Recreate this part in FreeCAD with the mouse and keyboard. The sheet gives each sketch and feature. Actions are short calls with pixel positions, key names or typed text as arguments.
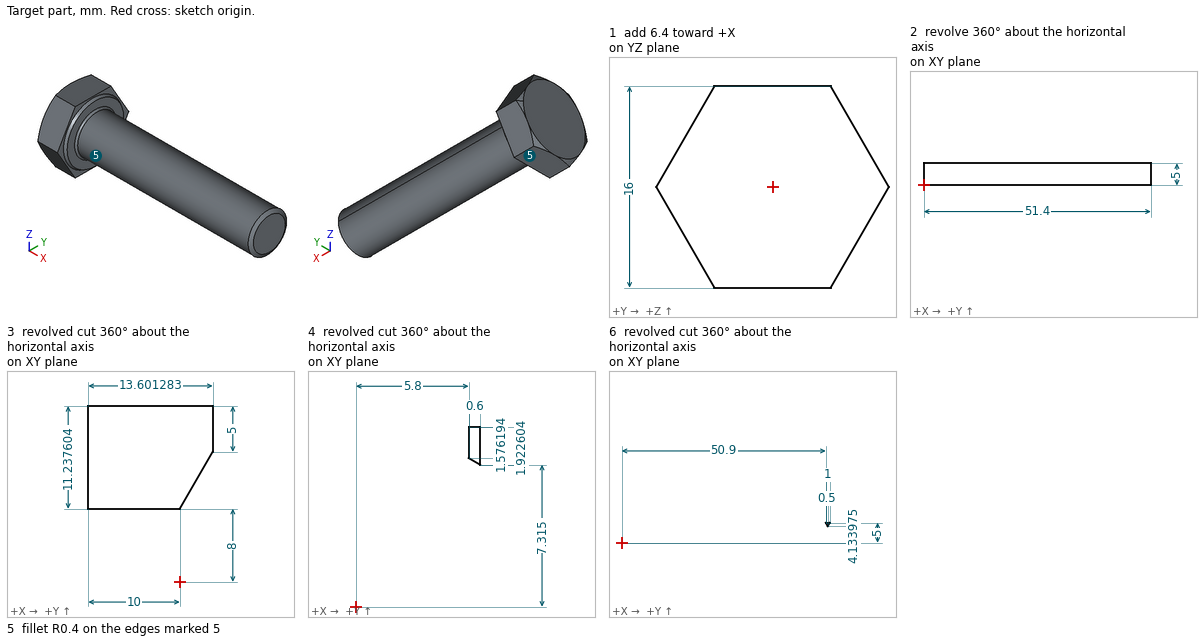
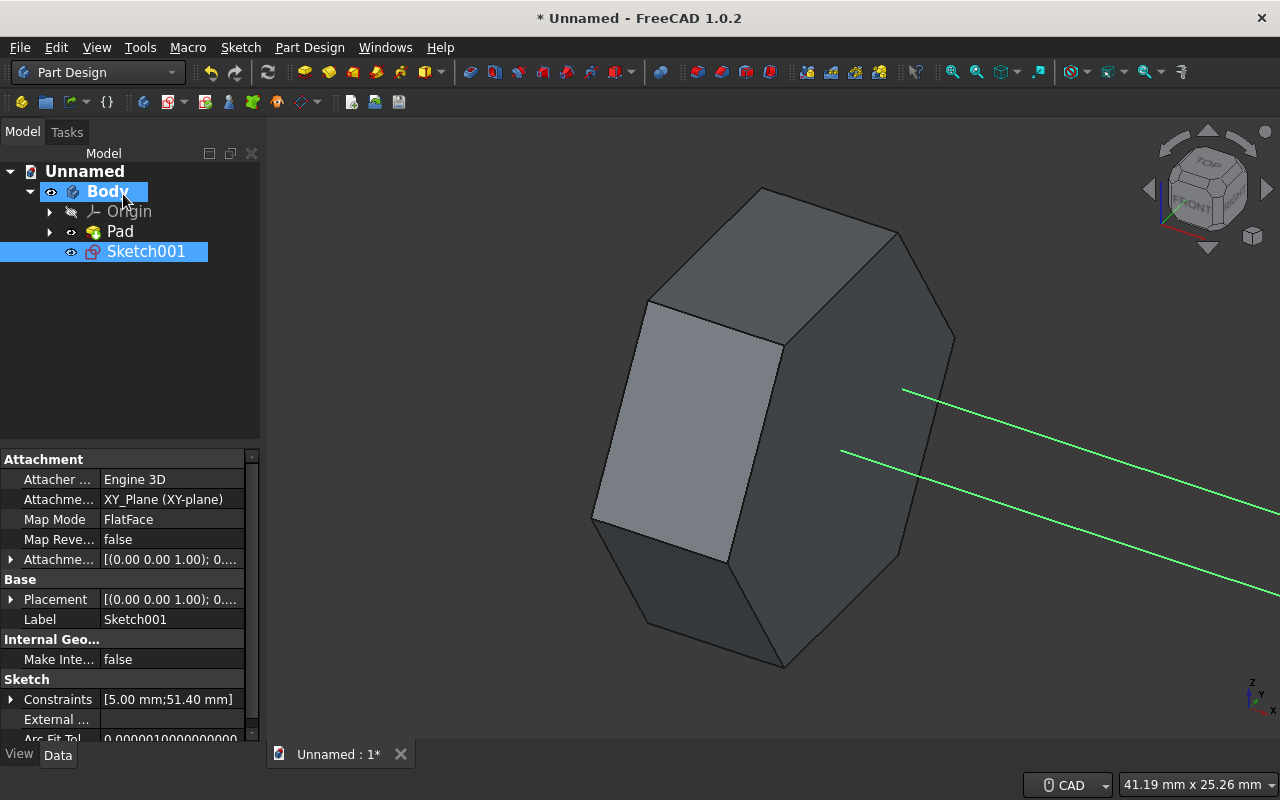
click(330, 72)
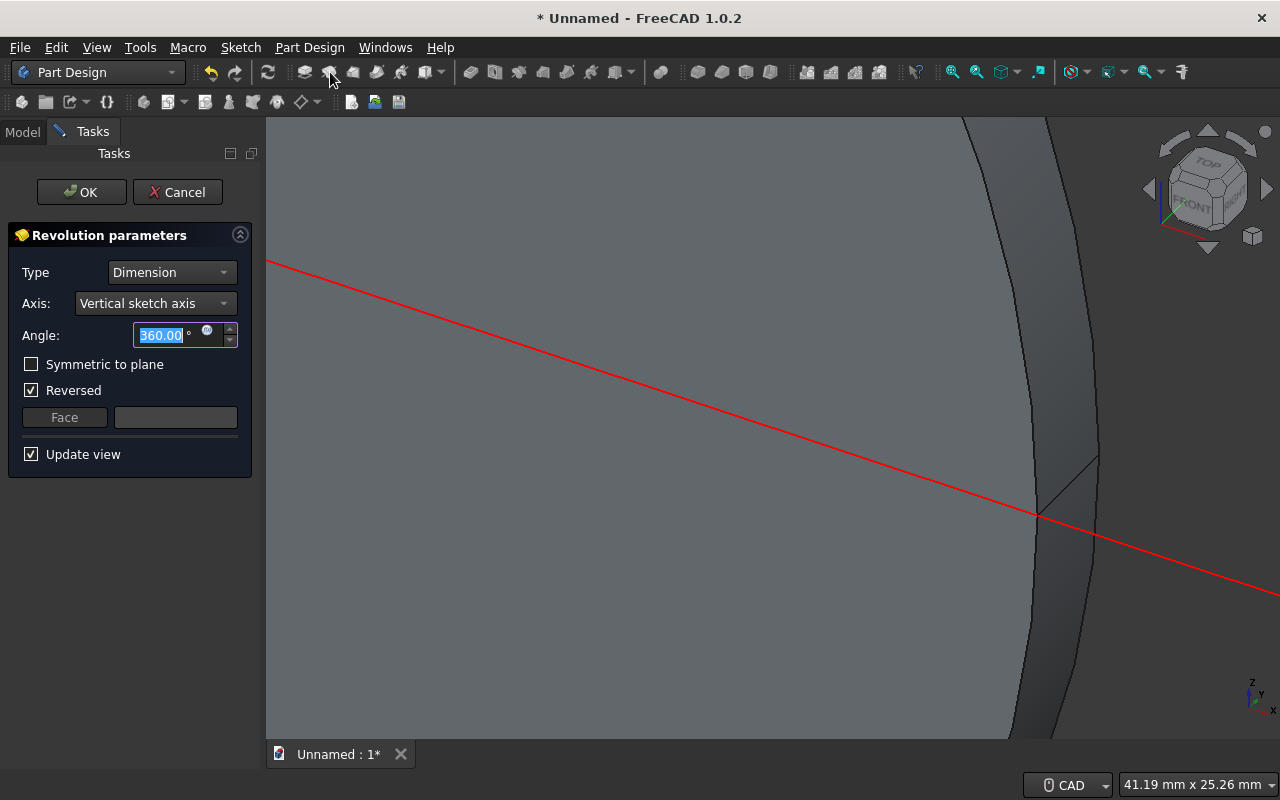
click(156, 304)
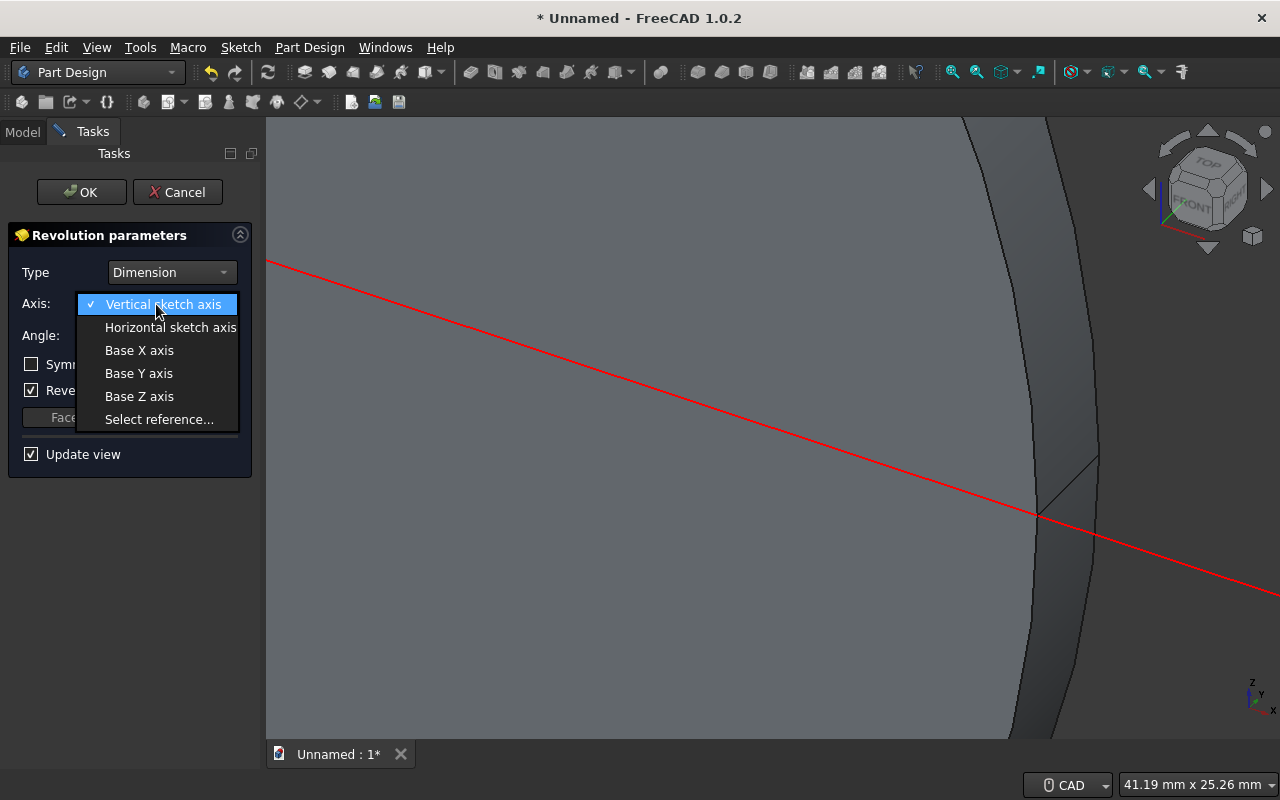
click(156, 328)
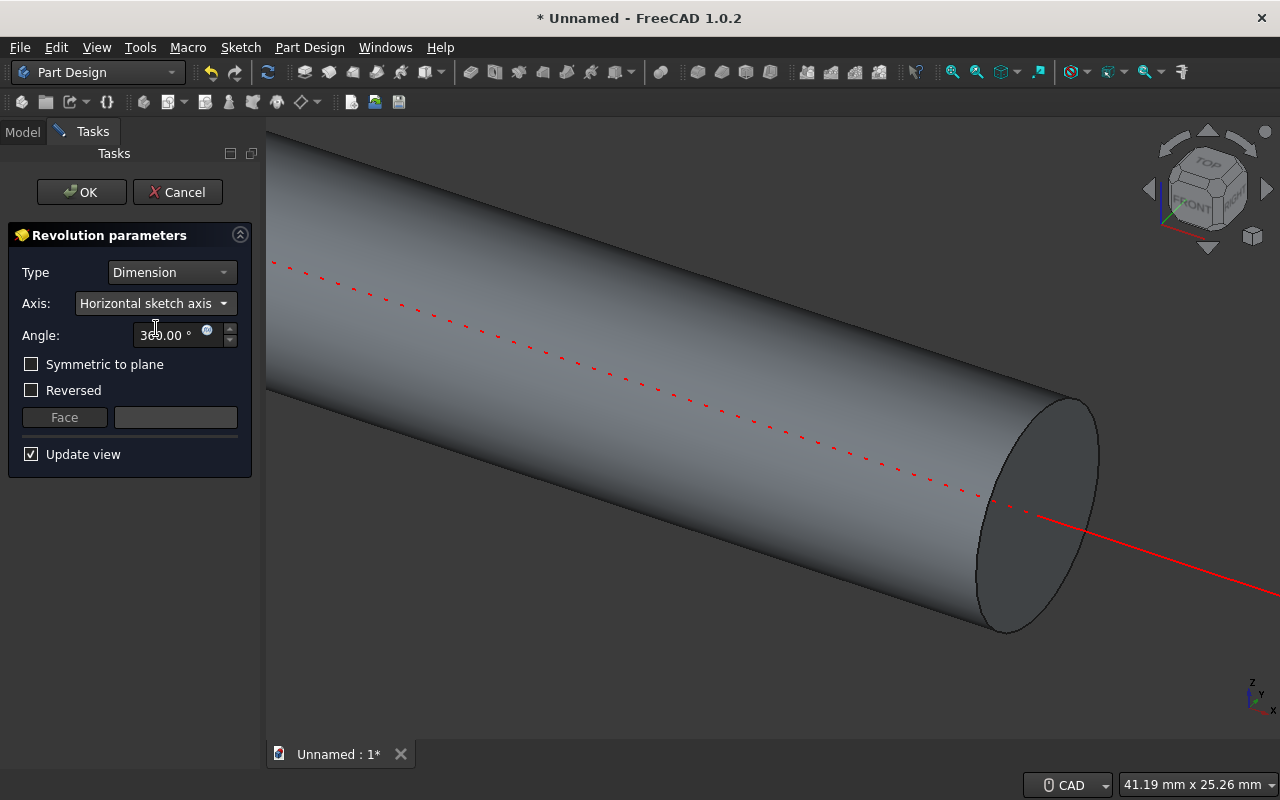
click(82, 192)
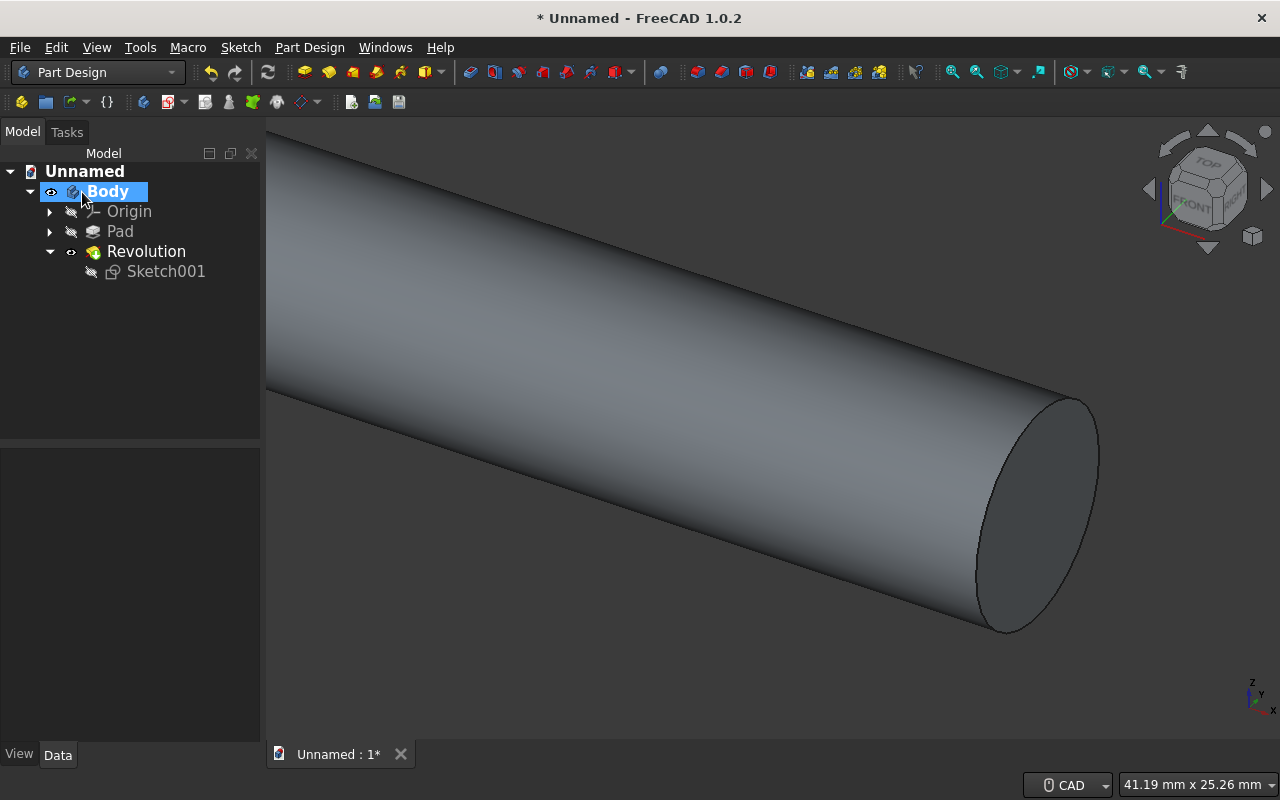
click(954, 72)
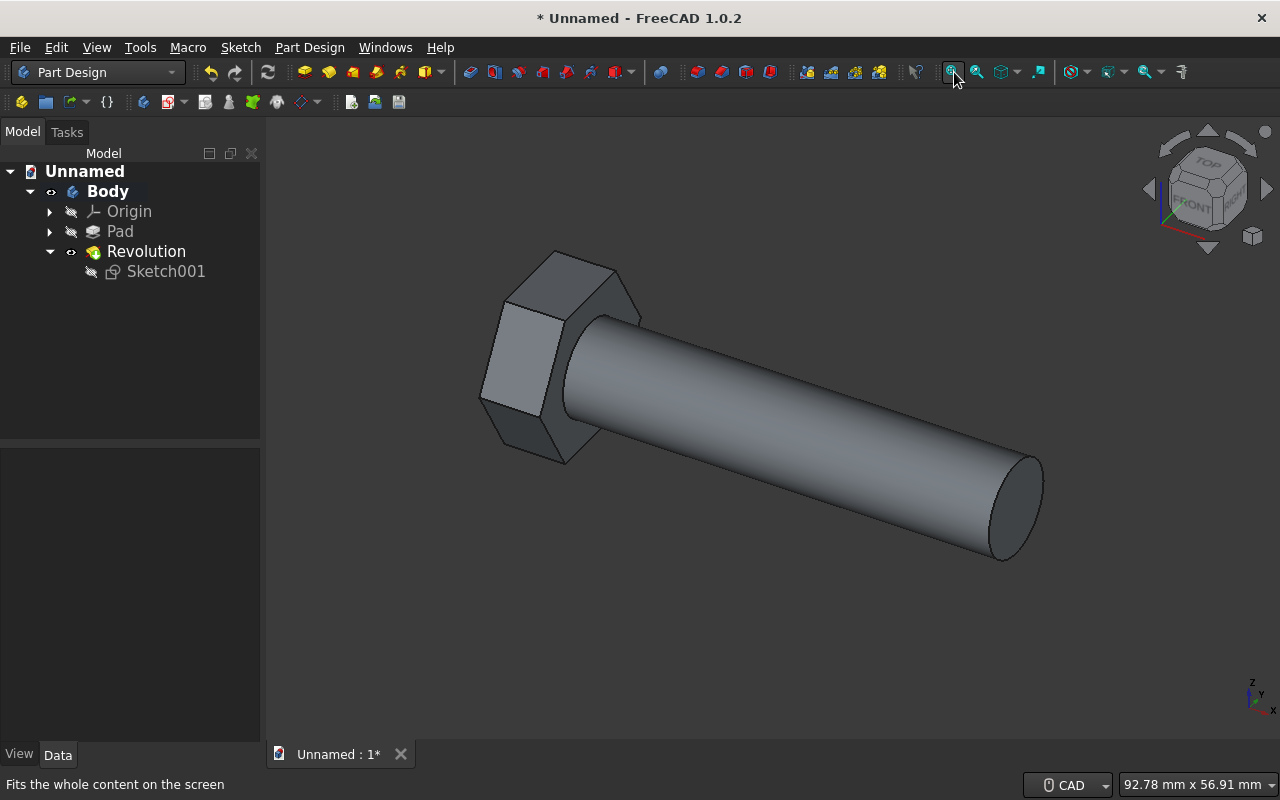
click(168, 102)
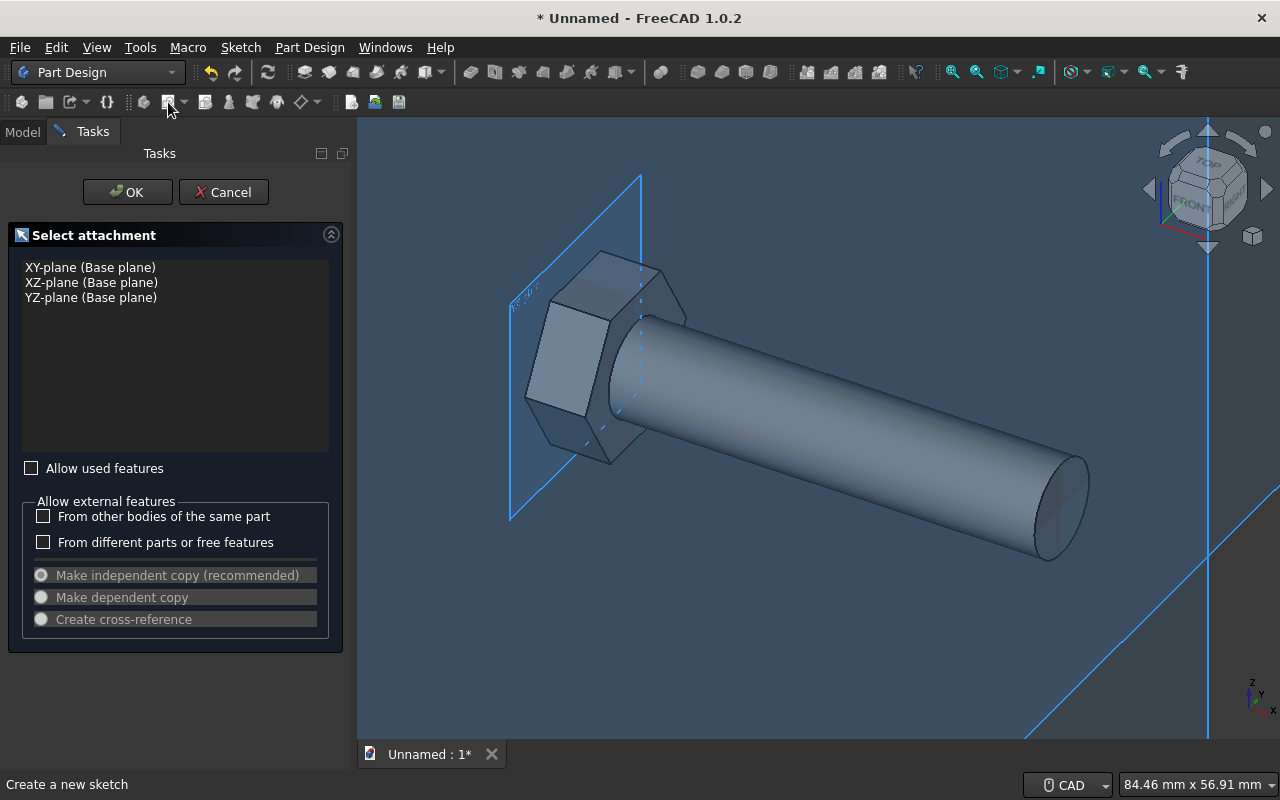
click(82, 268)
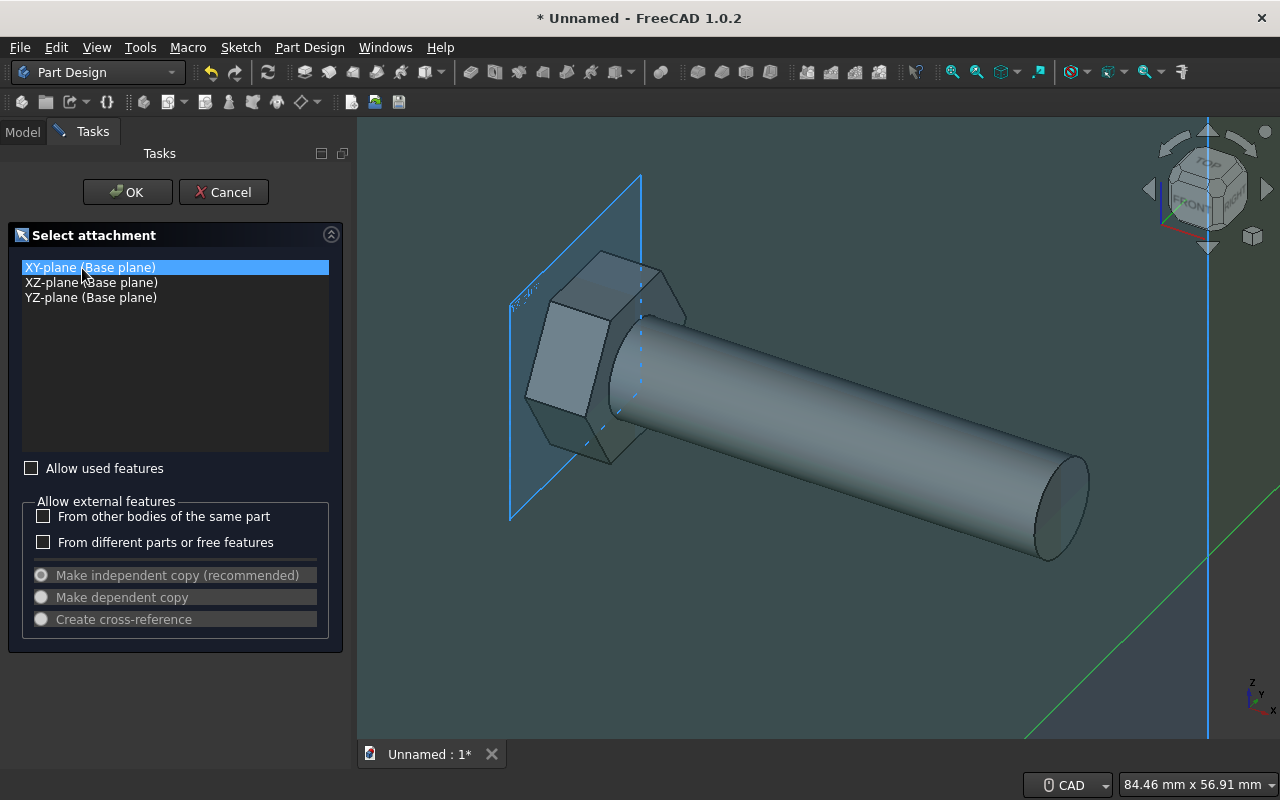
click(128, 192)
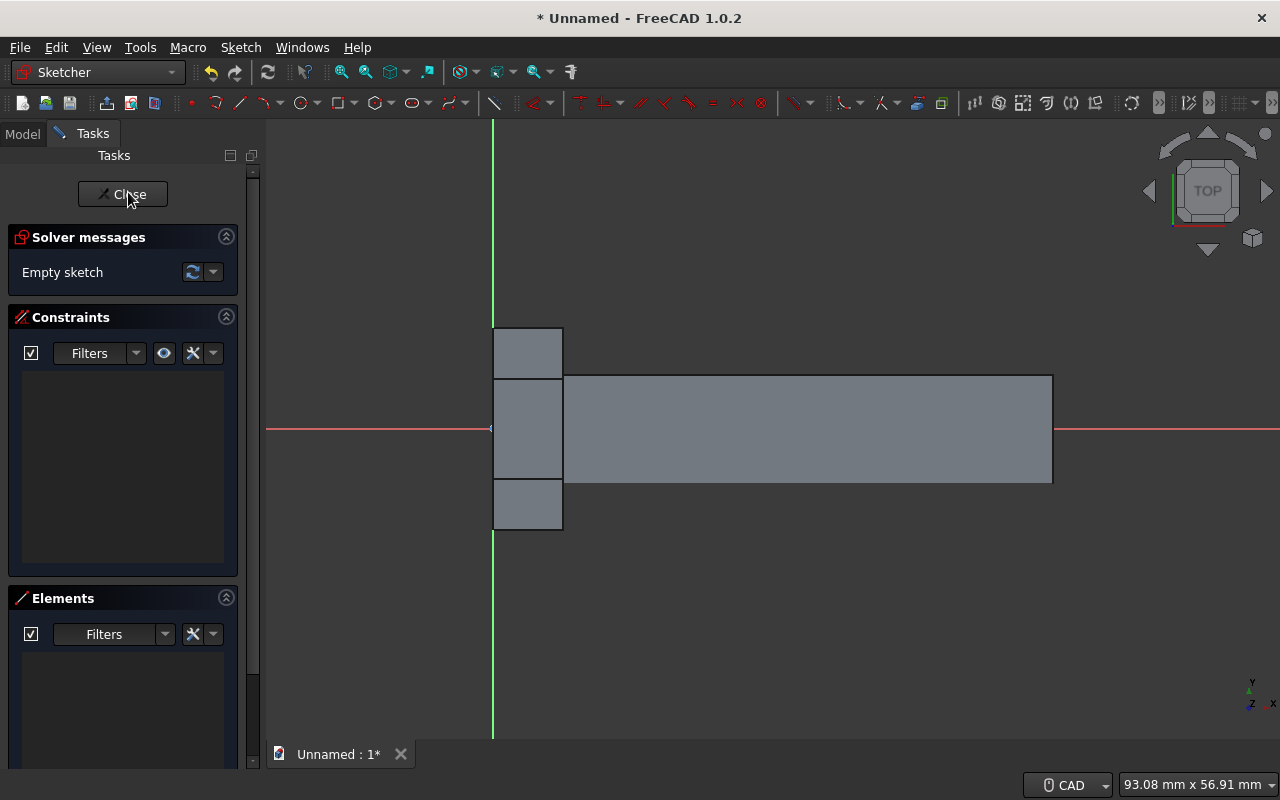
click(156, 104)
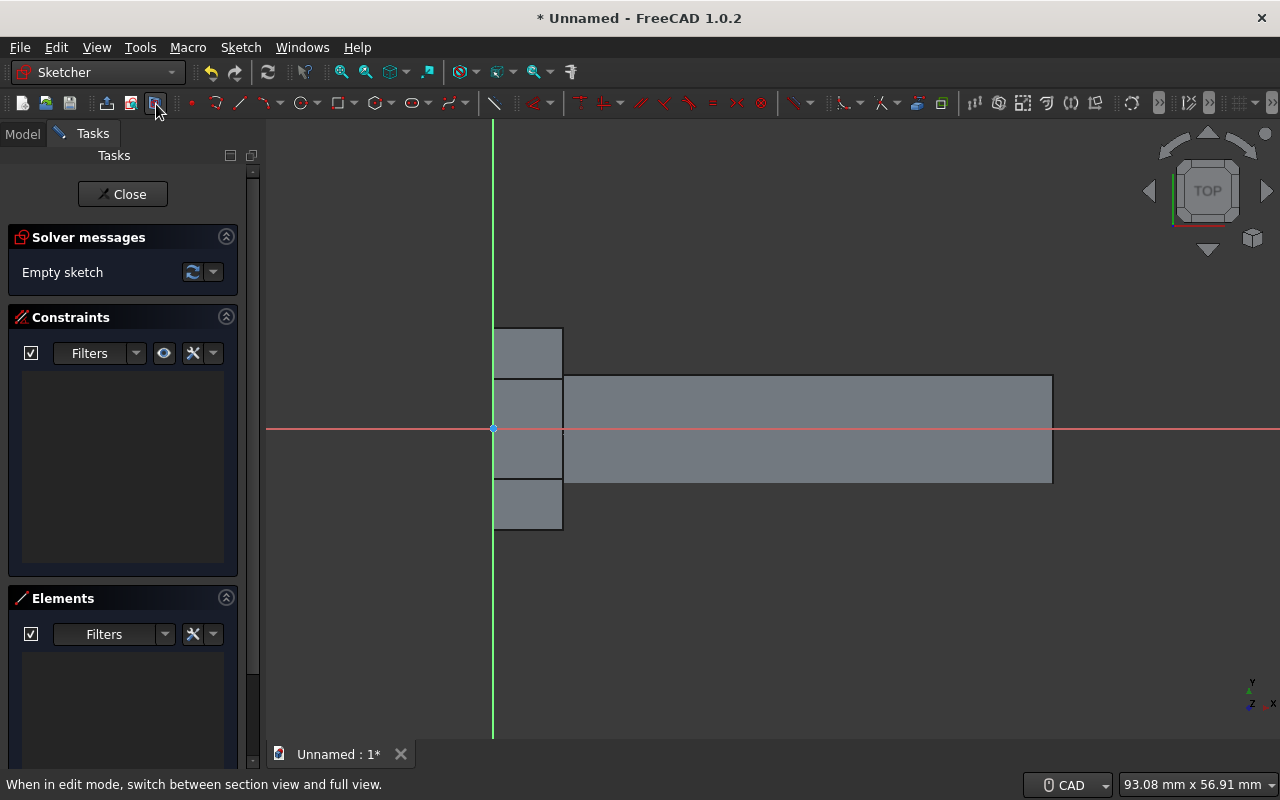
scroll(294, 197, up, 3)